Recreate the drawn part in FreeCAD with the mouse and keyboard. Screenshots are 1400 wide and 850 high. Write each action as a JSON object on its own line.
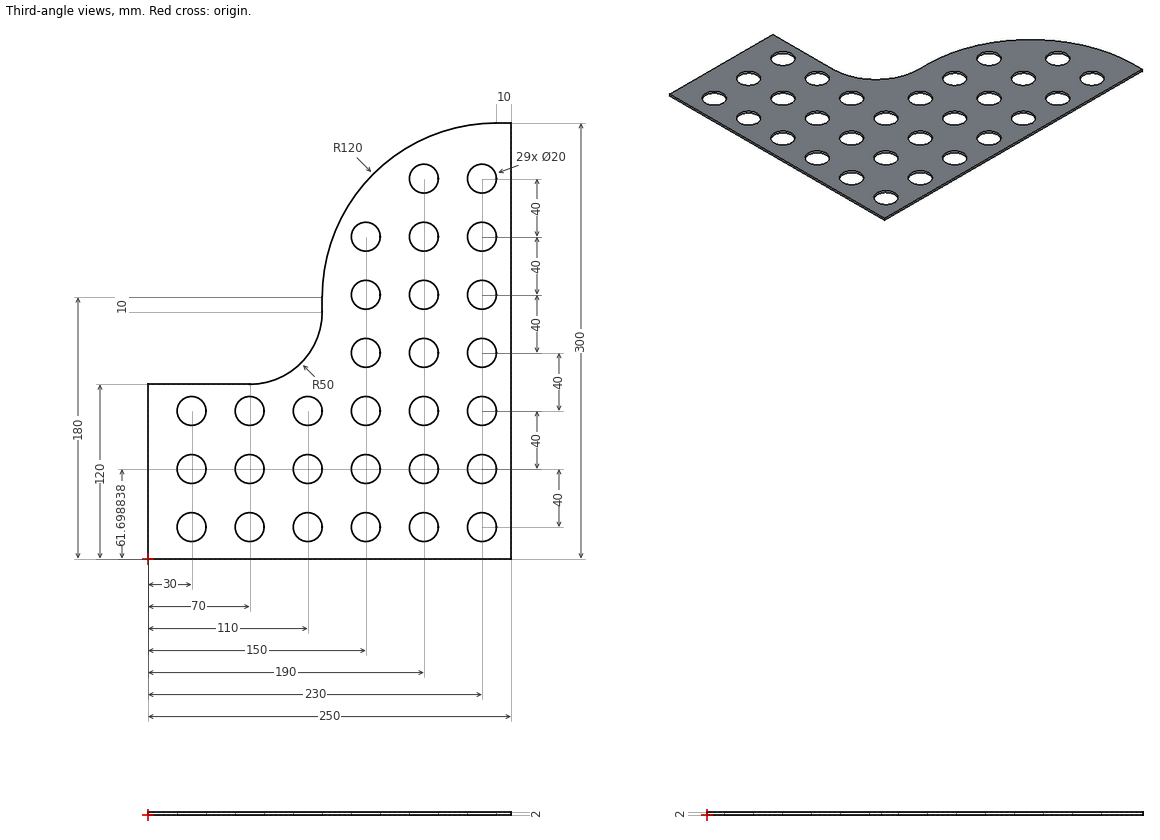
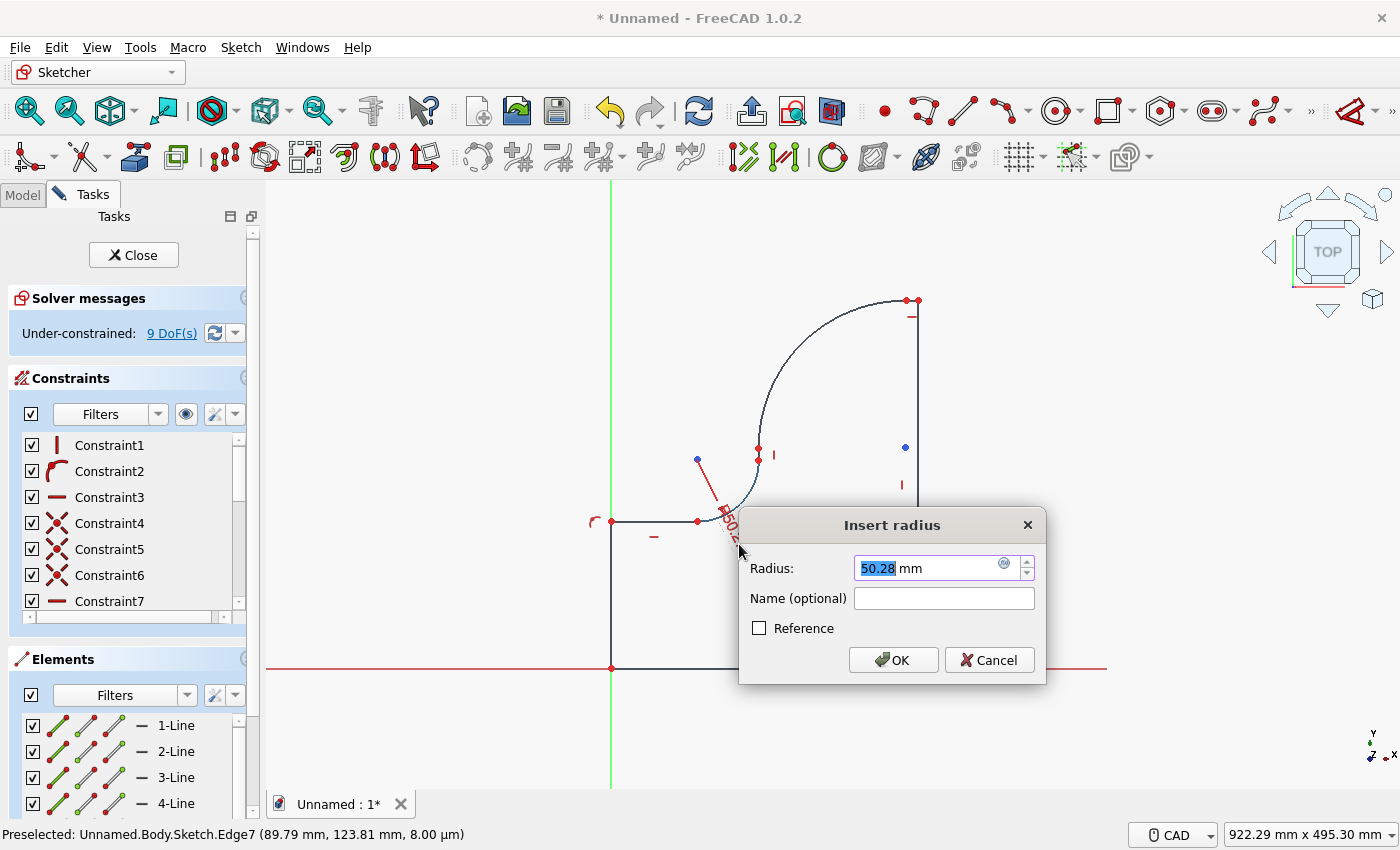
{"action": "type", "text": "50"}
{"action": "key", "text": "Return"}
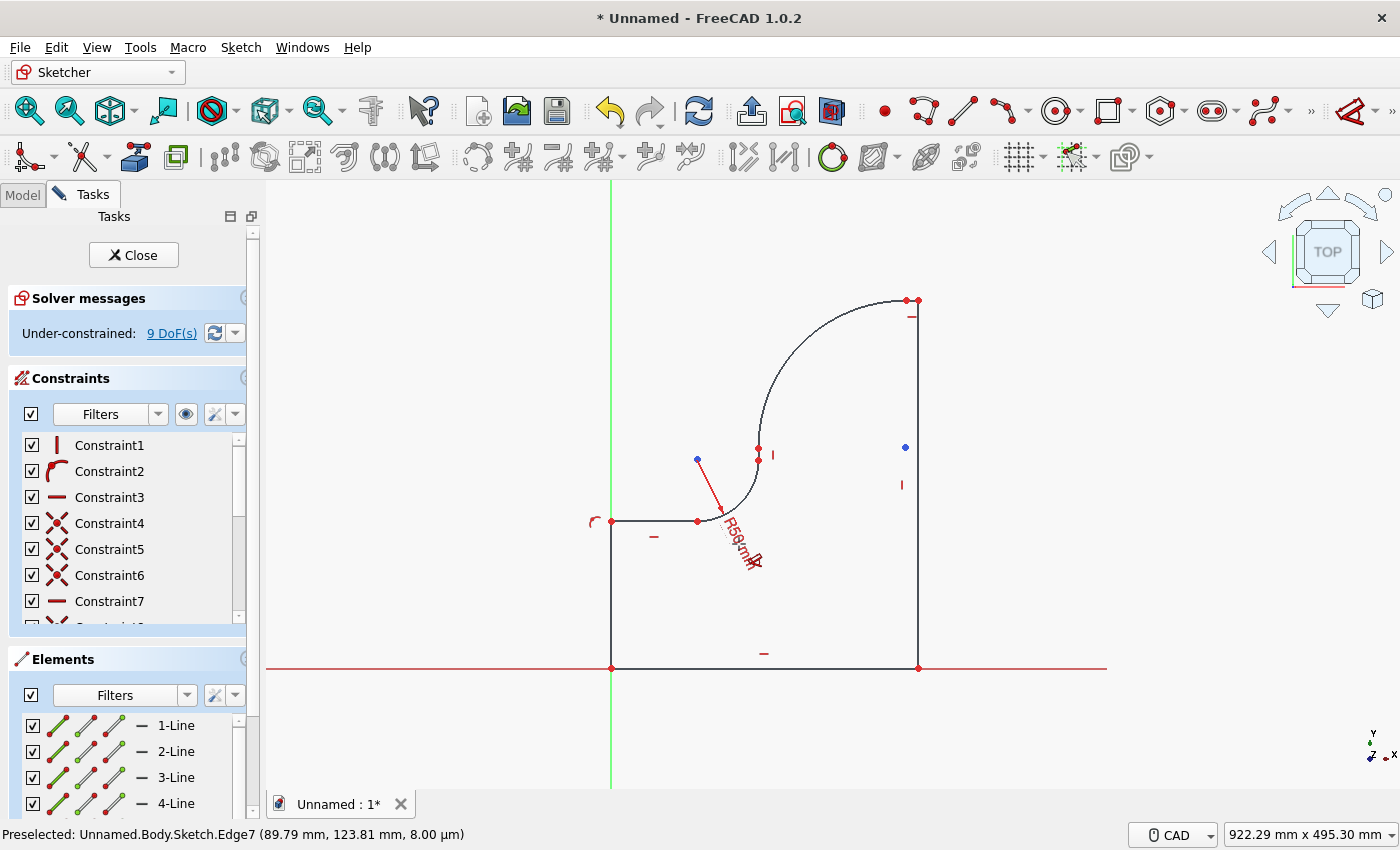
{"action": "left_click", "coordinate": [839, 317]}
{"action": "left_click", "coordinate": [825, 288]}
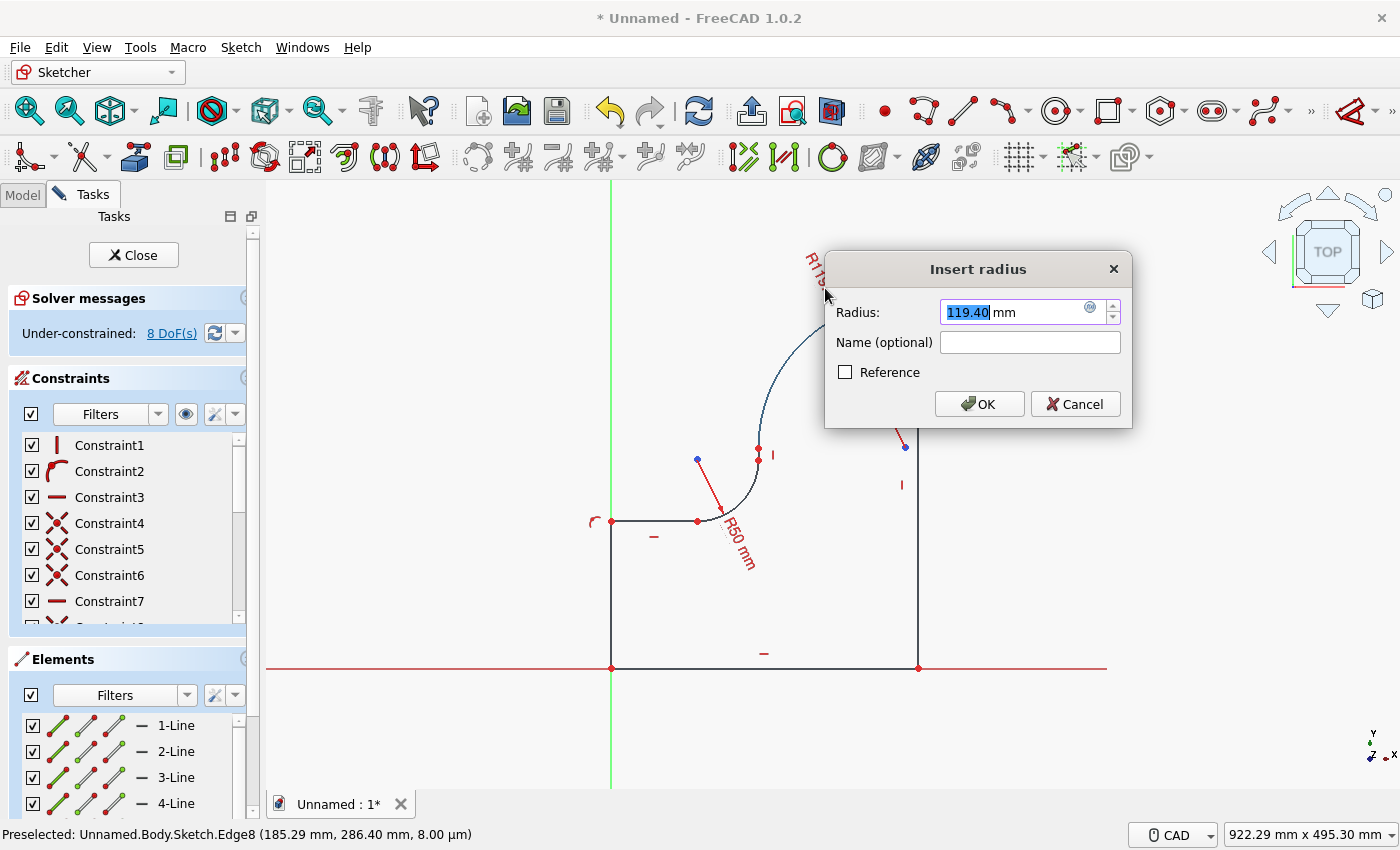
{"action": "type", "text": "120"}
{"action": "key", "text": "Return"}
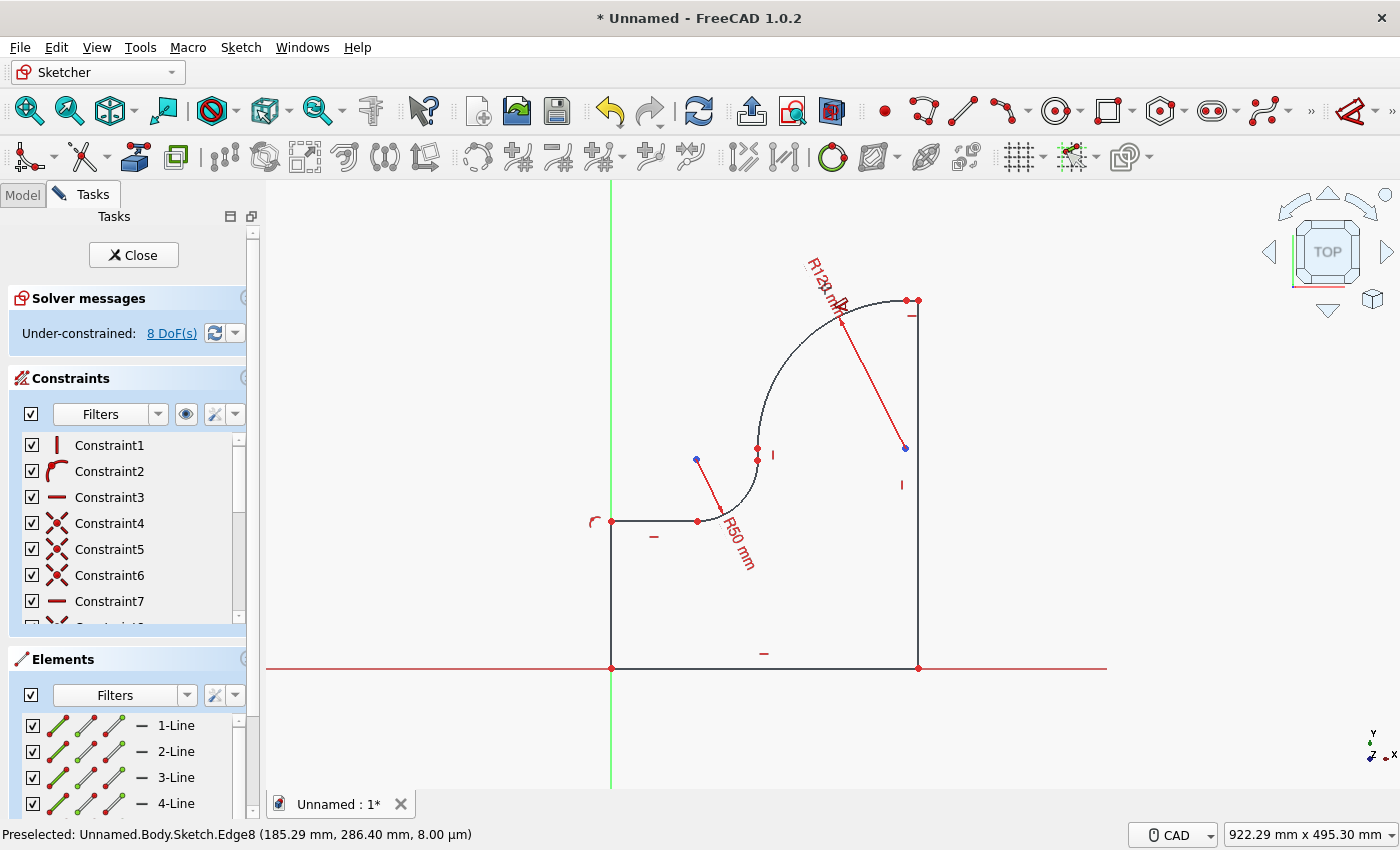
{"action": "scroll", "coordinate": [758, 455], "scroll_direction": "up", "scroll_amount": 6}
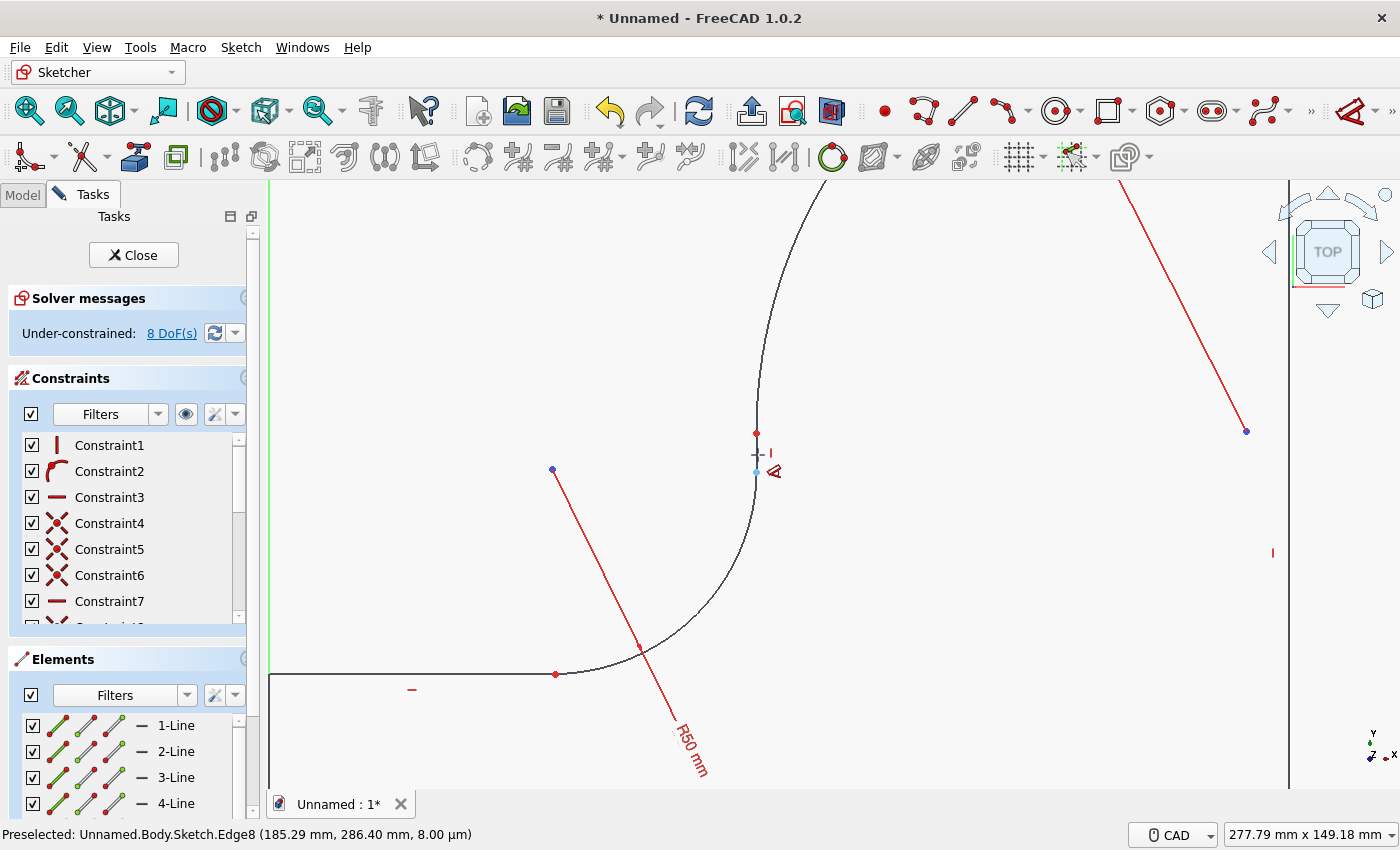
{"action": "left_click", "coordinate": [757, 453]}
{"action": "left_click", "coordinate": [723, 453]}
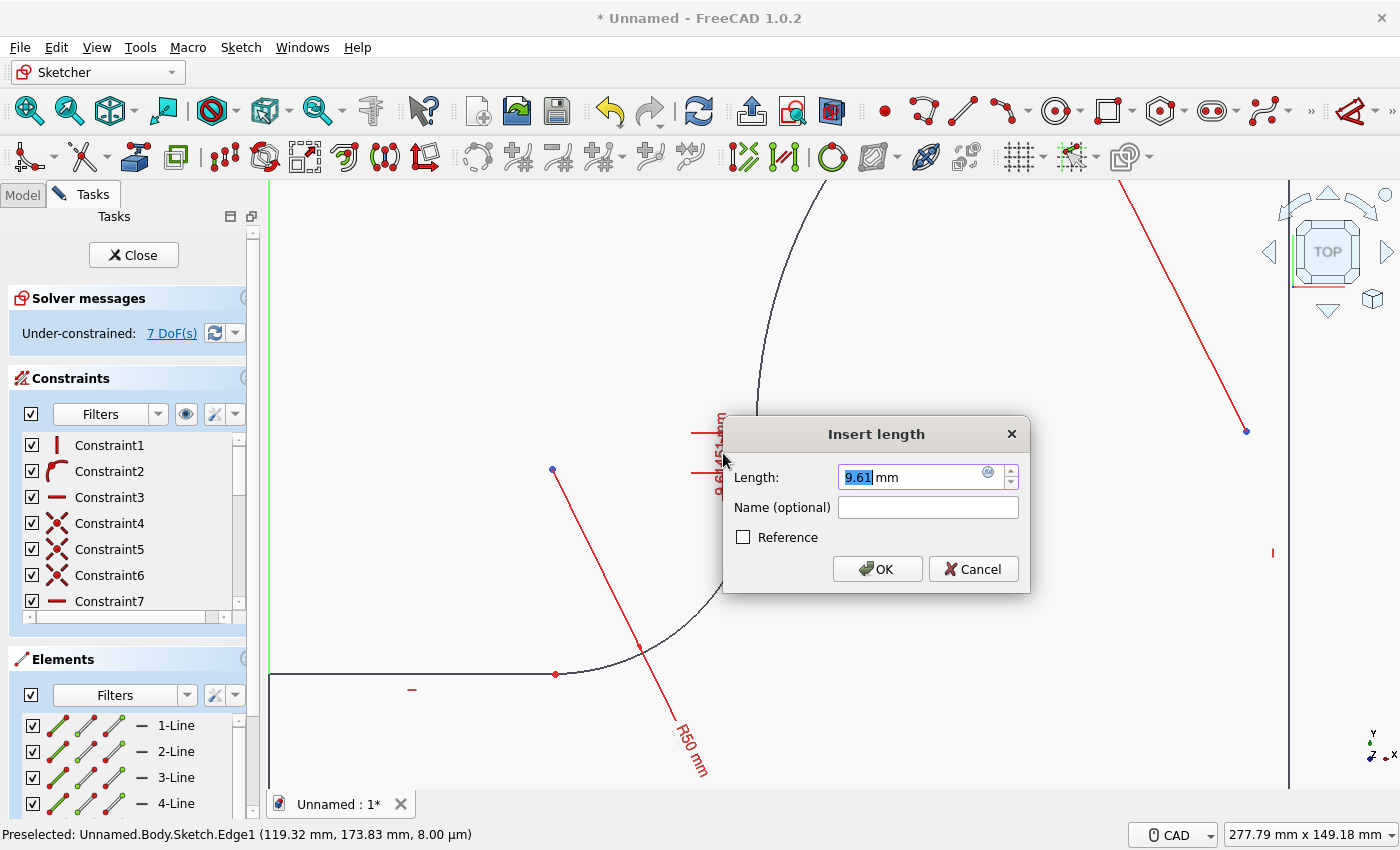
{"action": "type", "text": "10"}
{"action": "key", "text": "Return"}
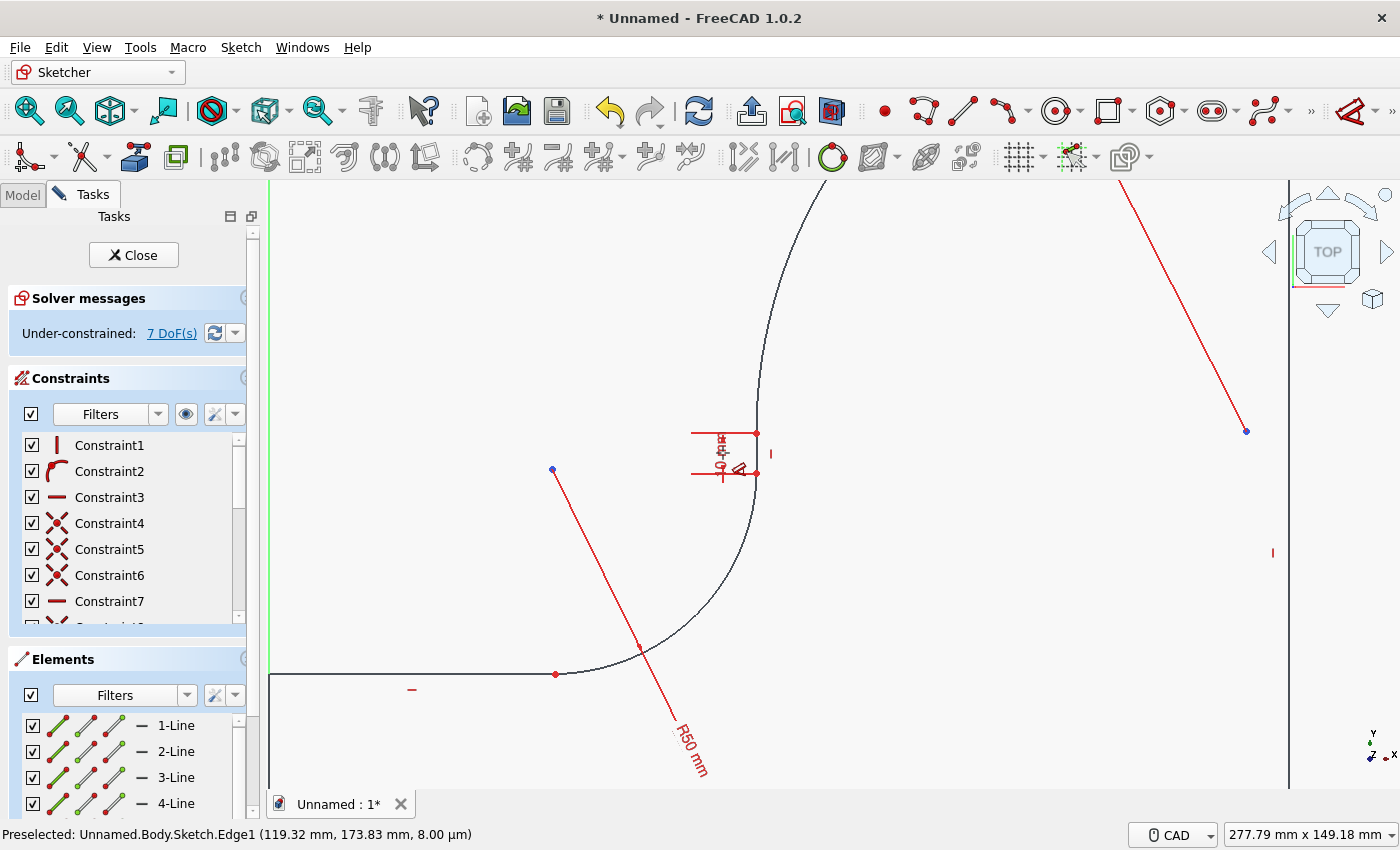
{"action": "left_click", "coordinate": [470, 674]}
{"action": "left_click", "coordinate": [425, 708]}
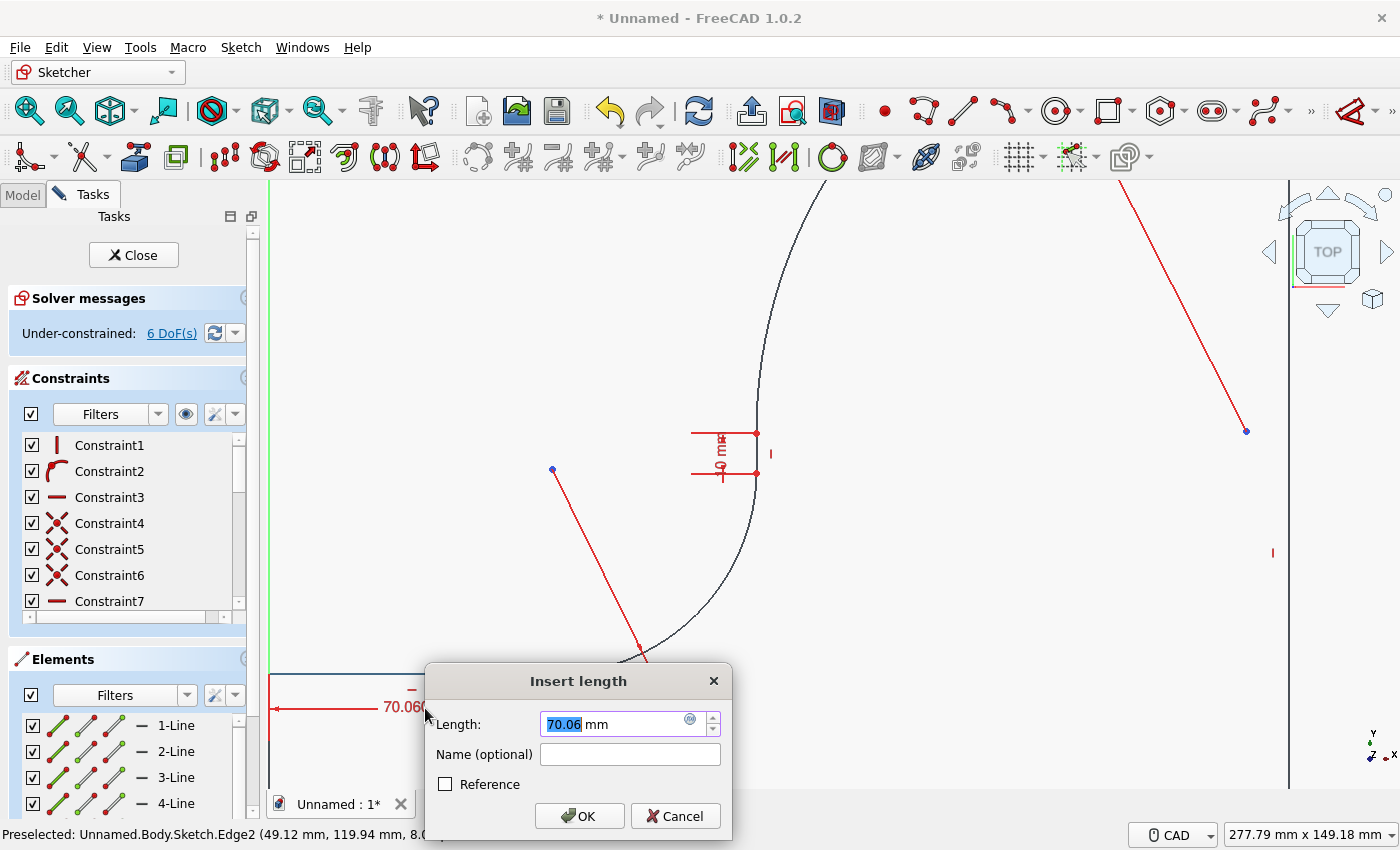
{"action": "type", "text": "70"}
{"action": "key", "text": "Return"}